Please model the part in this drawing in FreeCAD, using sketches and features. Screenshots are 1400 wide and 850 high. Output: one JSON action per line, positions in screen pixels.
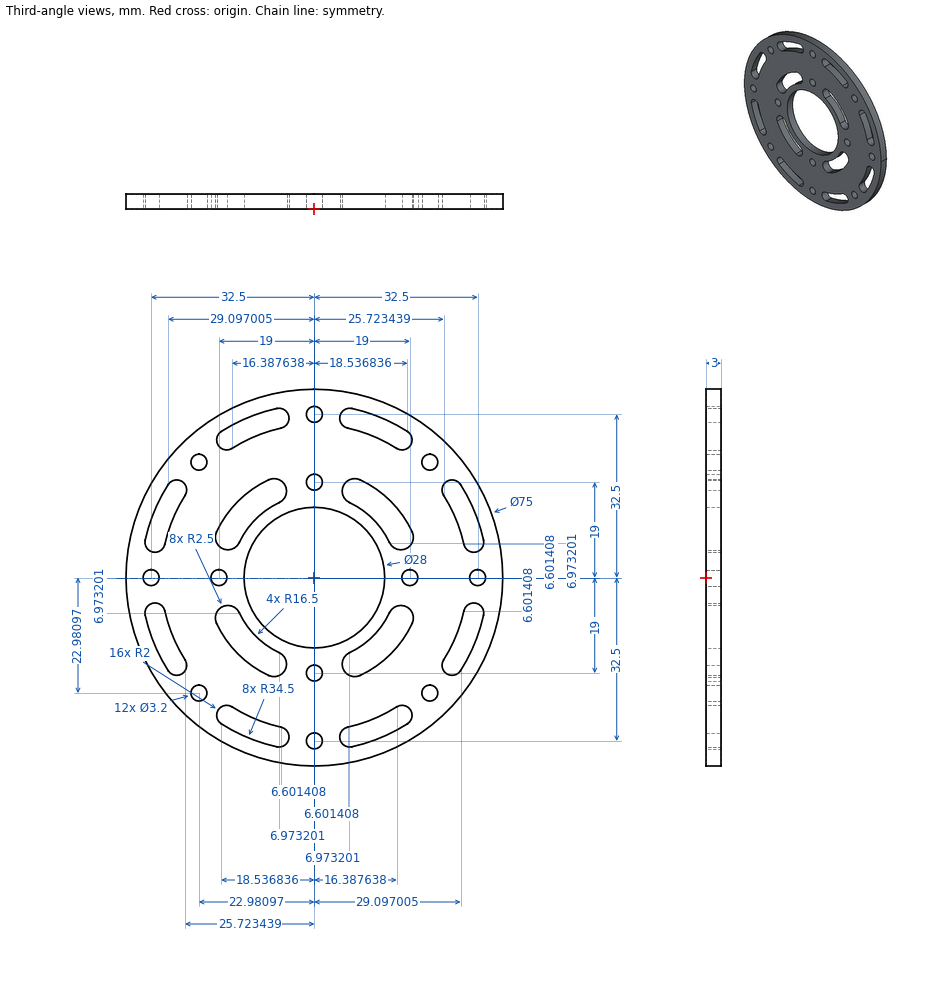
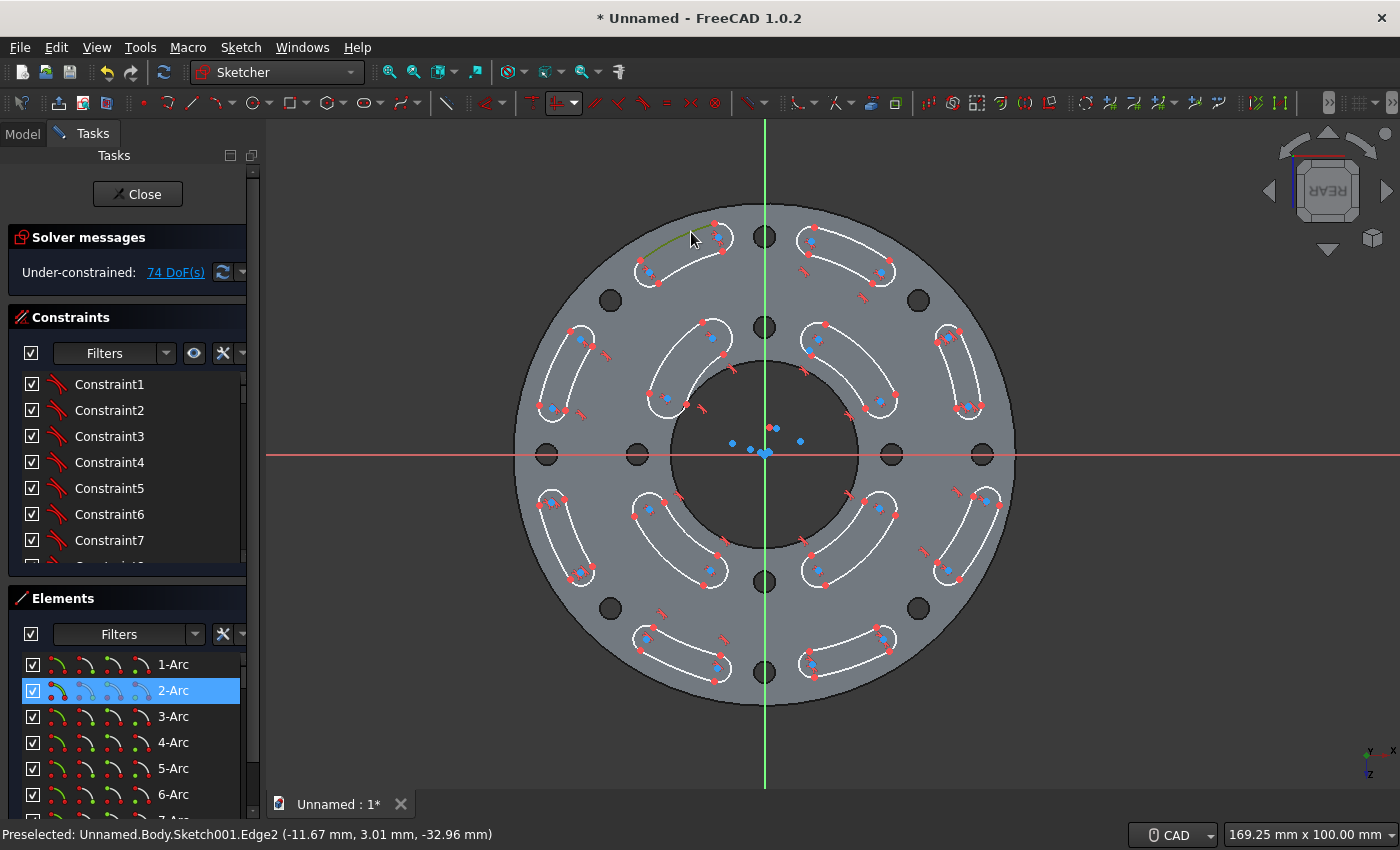
{"action": "left_click", "coordinate": [673, 638]}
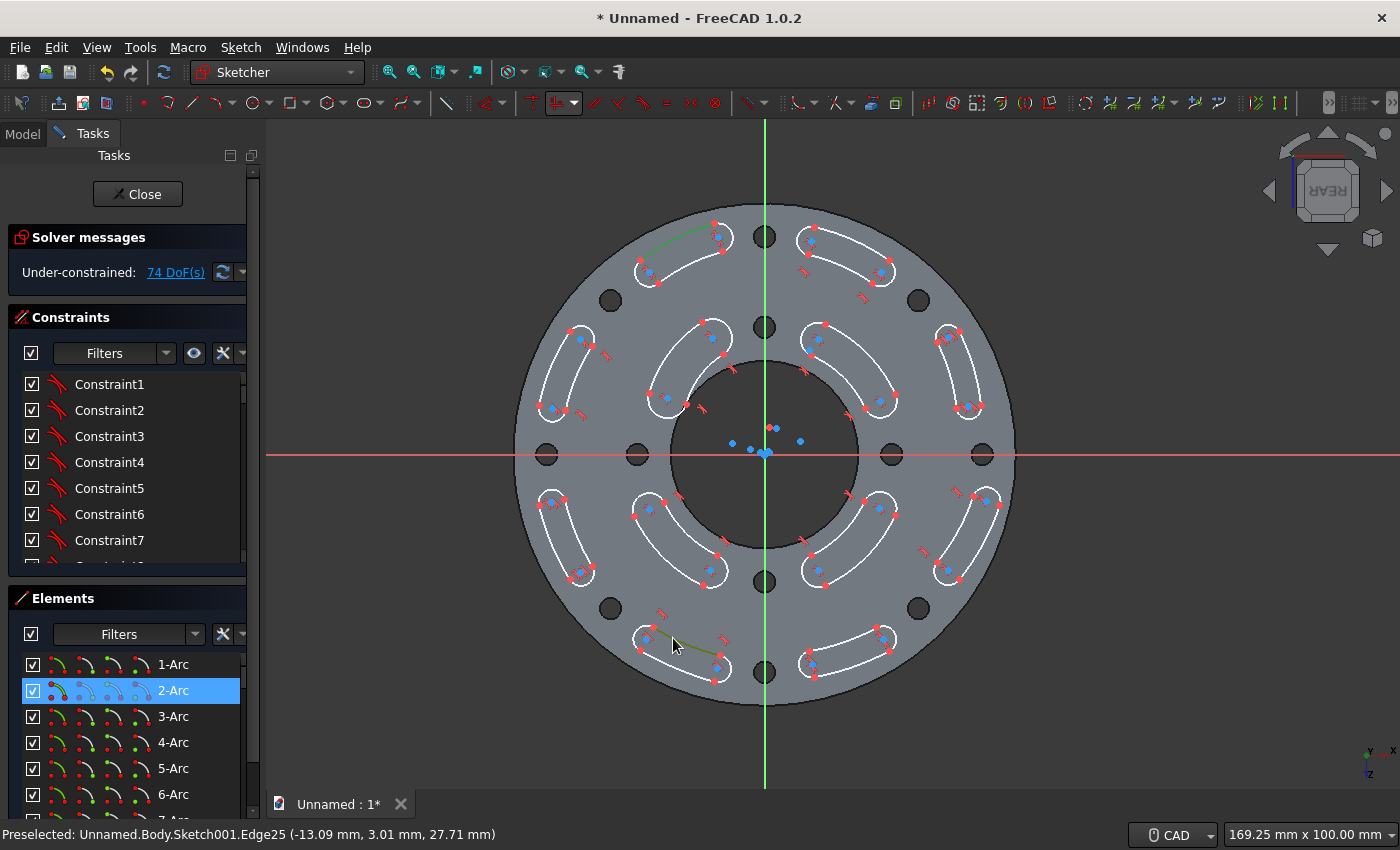
{"action": "left_click", "coordinate": [532, 104]}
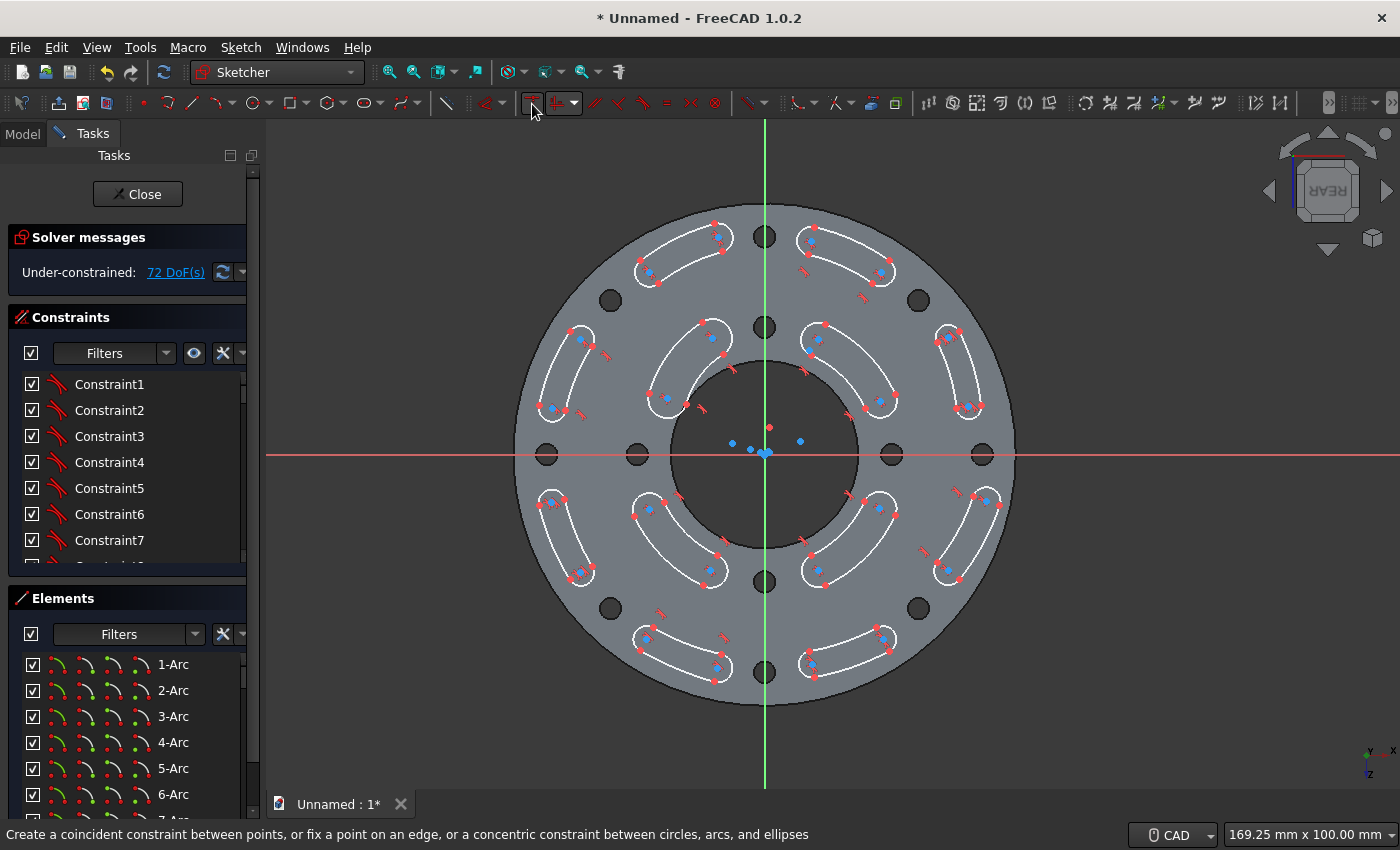
{"action": "left_click", "coordinate": [691, 232]}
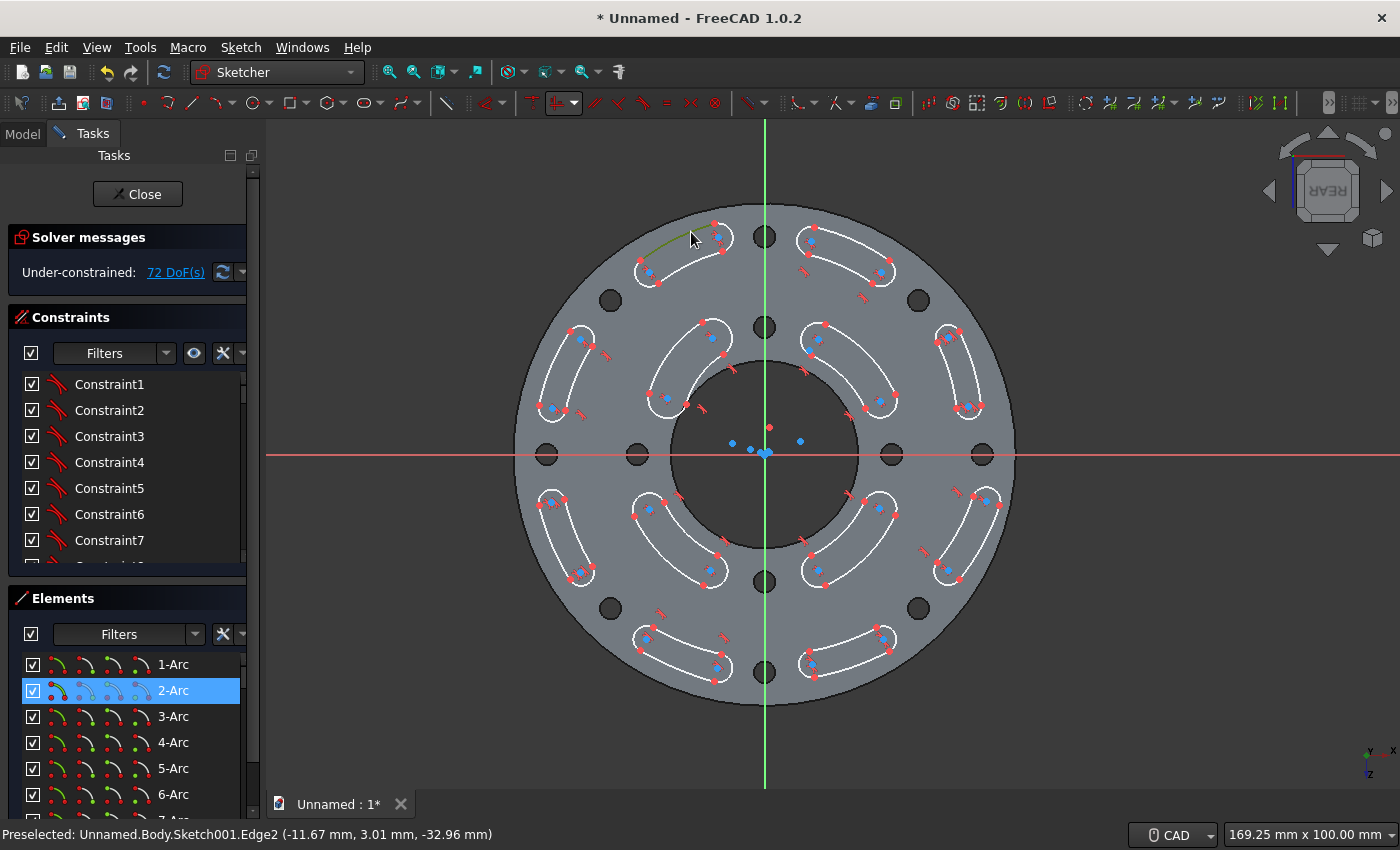
{"action": "left_click", "coordinate": [662, 662]}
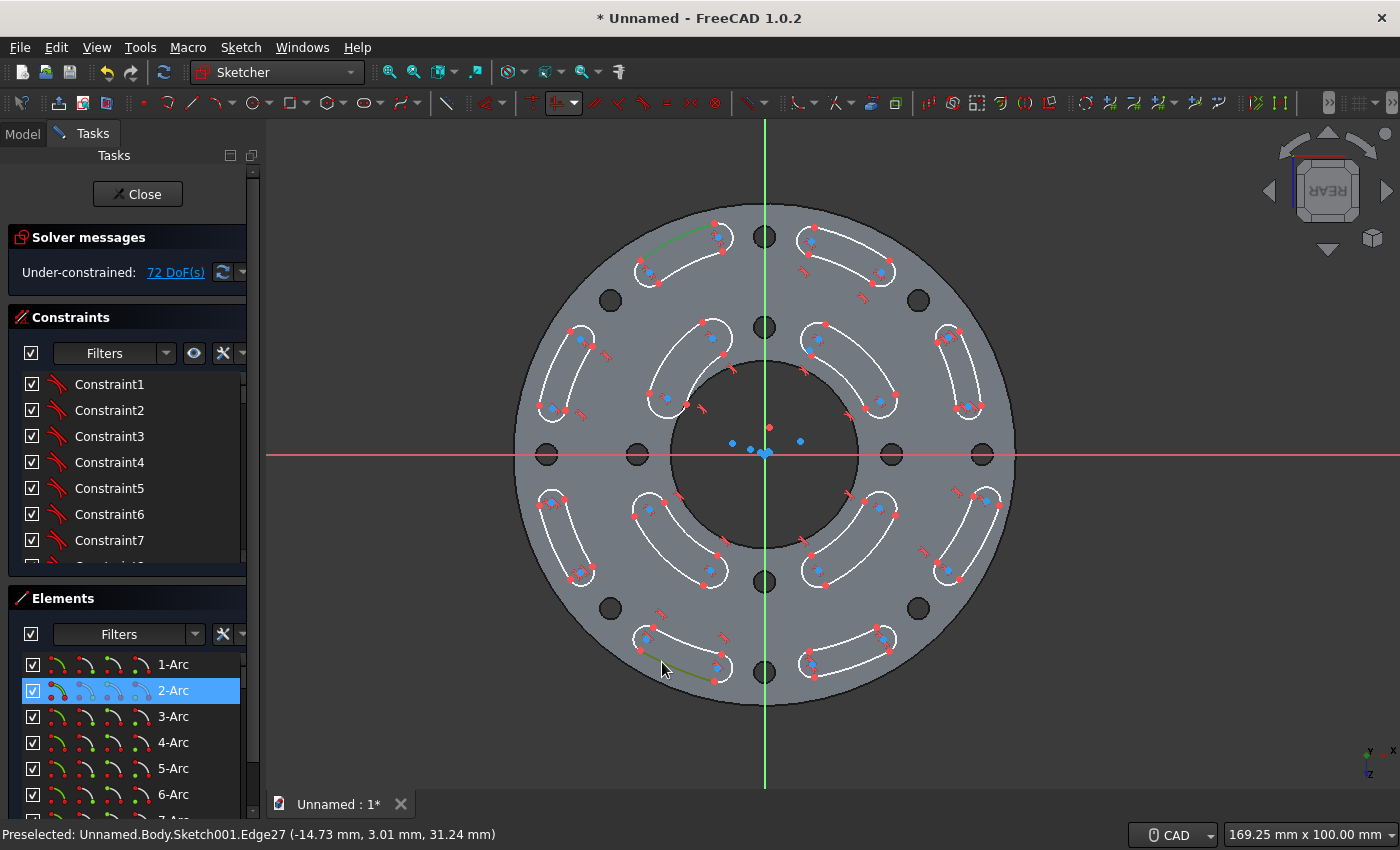
{"action": "left_click", "coordinate": [532, 104]}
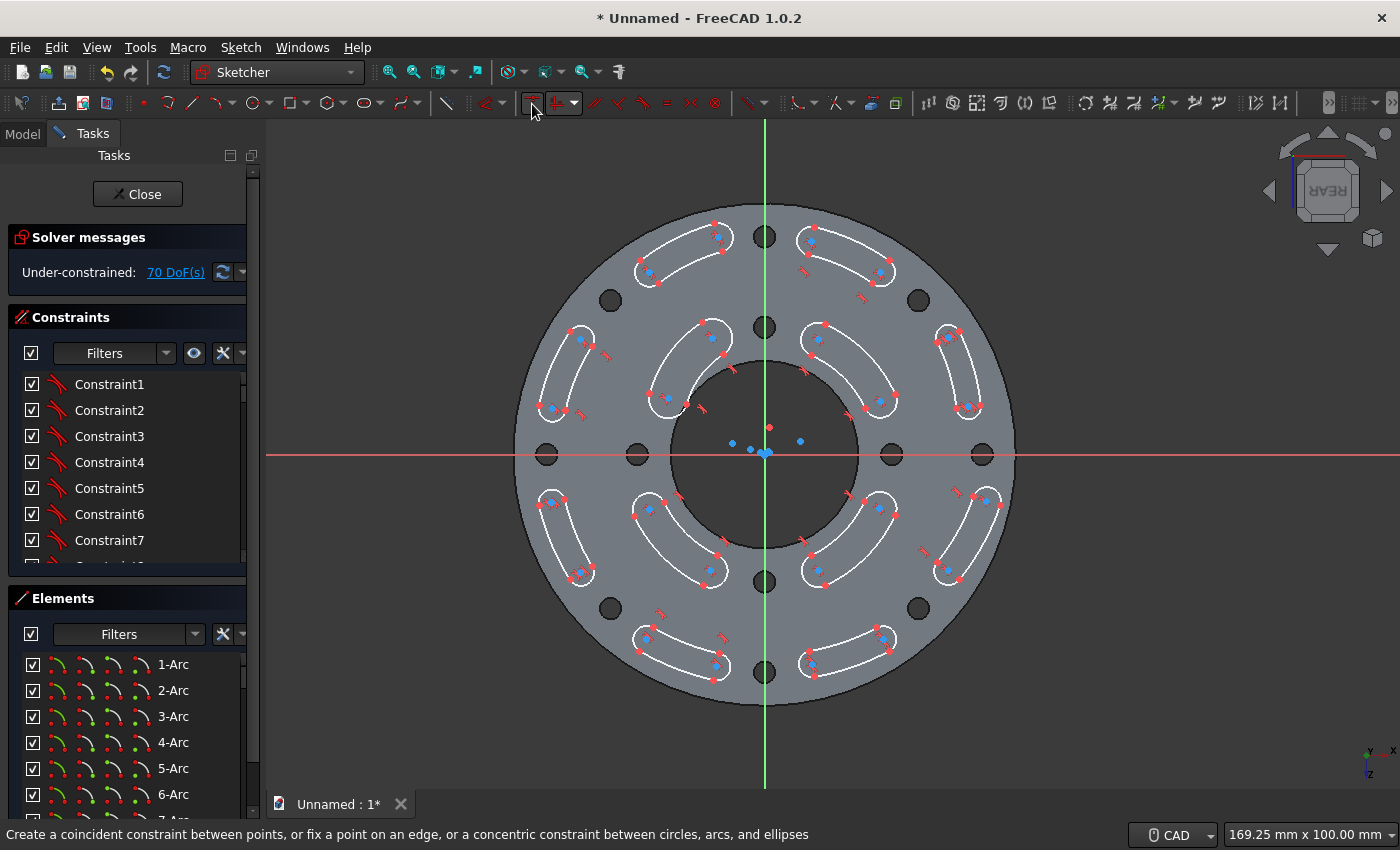
{"action": "left_click", "coordinate": [691, 232]}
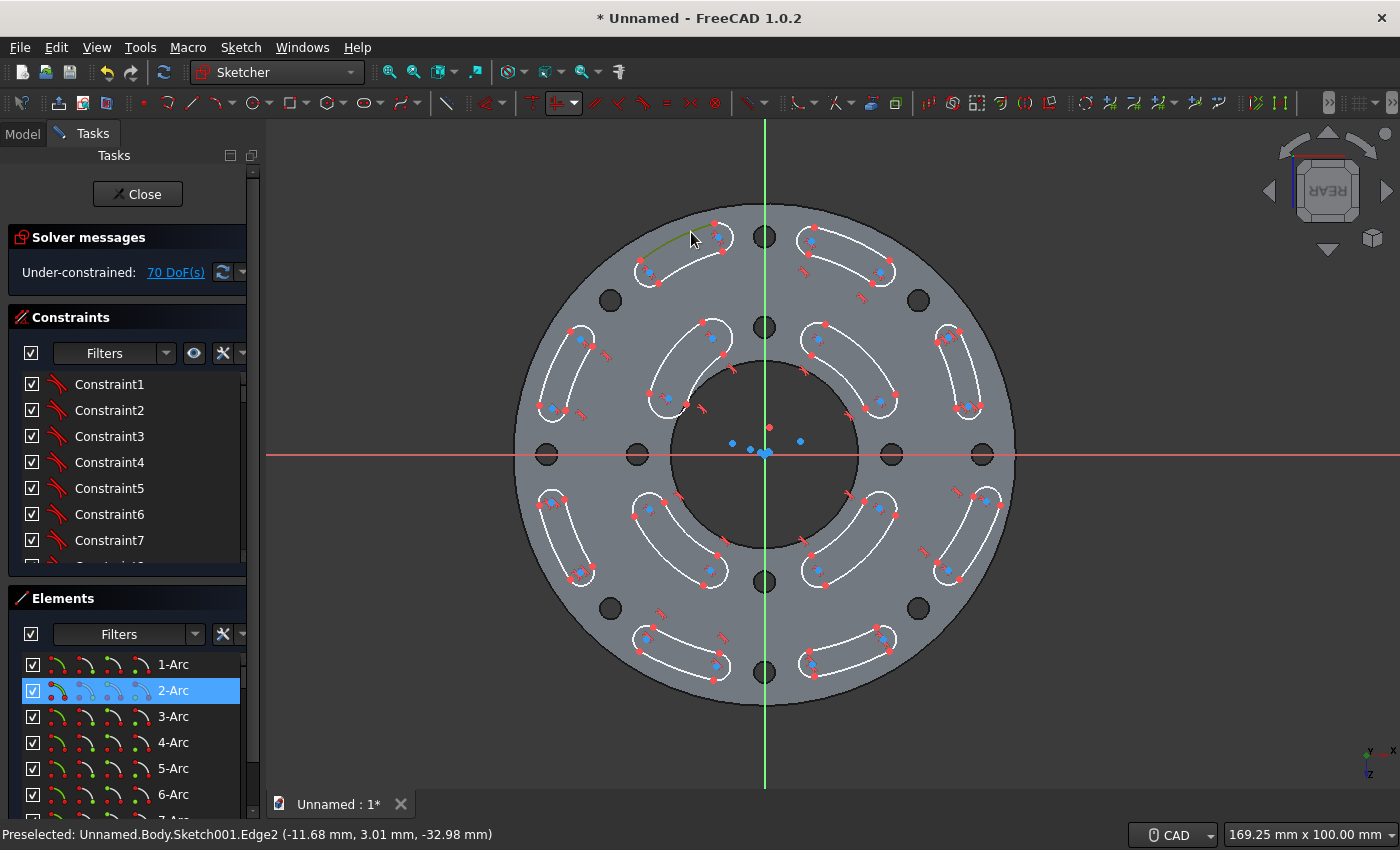
{"action": "left_click", "coordinate": [546, 529]}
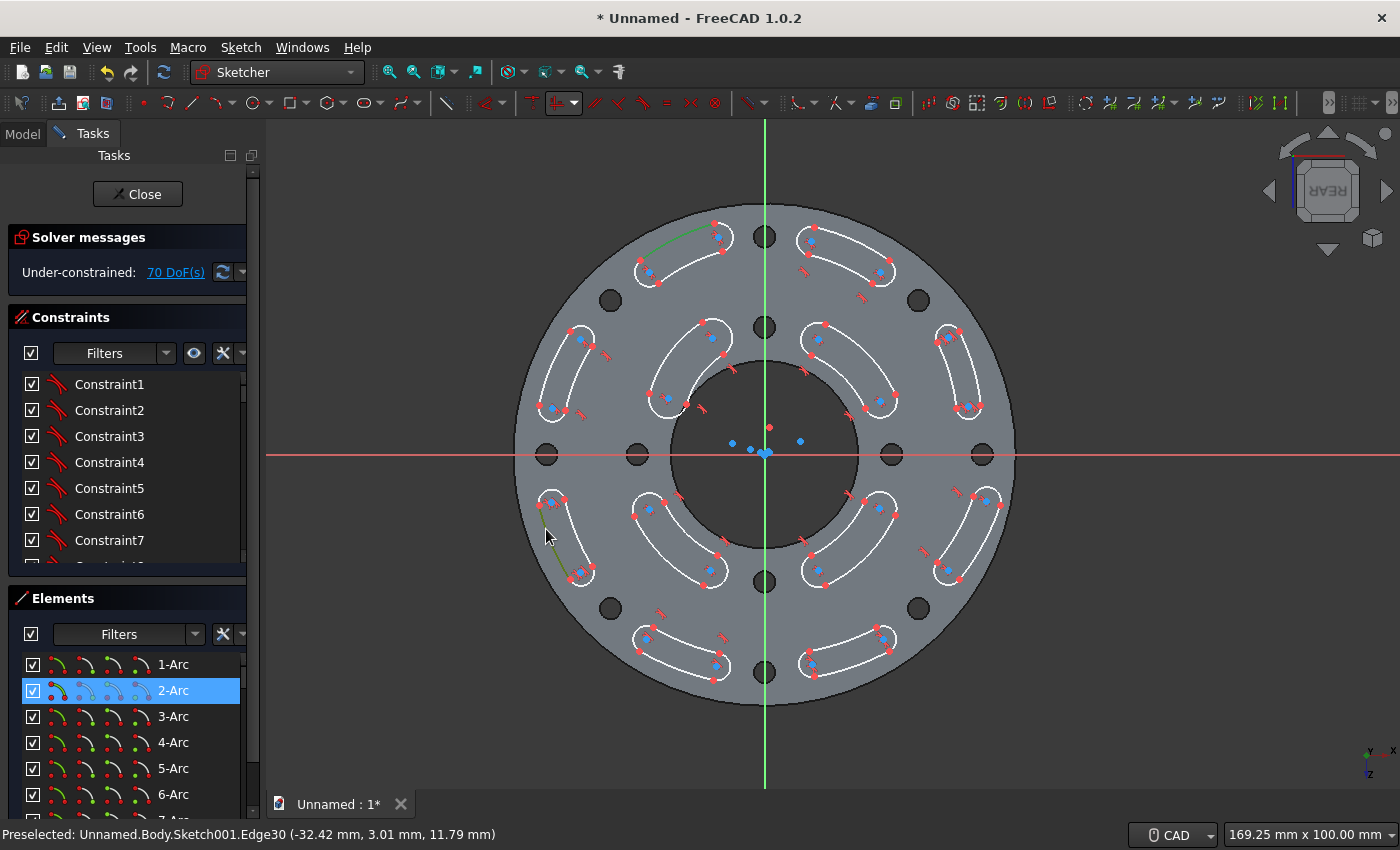
{"action": "left_click", "coordinate": [532, 104]}